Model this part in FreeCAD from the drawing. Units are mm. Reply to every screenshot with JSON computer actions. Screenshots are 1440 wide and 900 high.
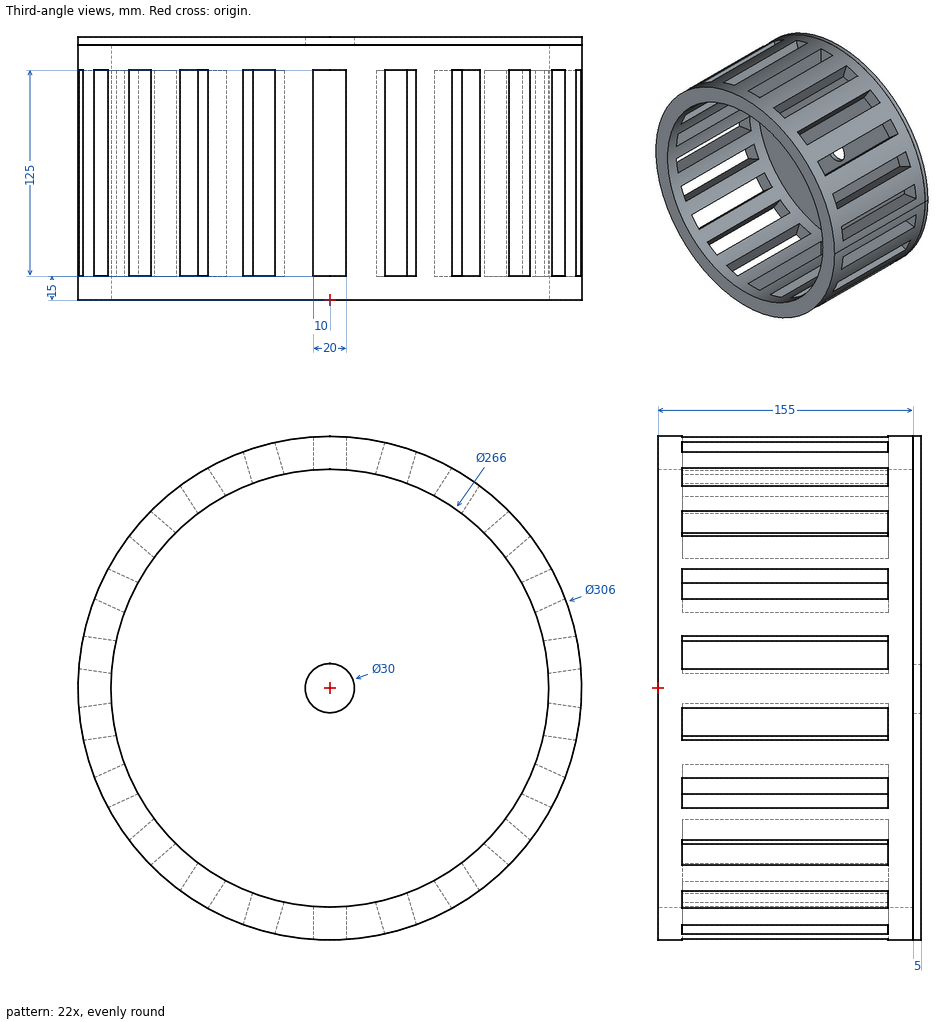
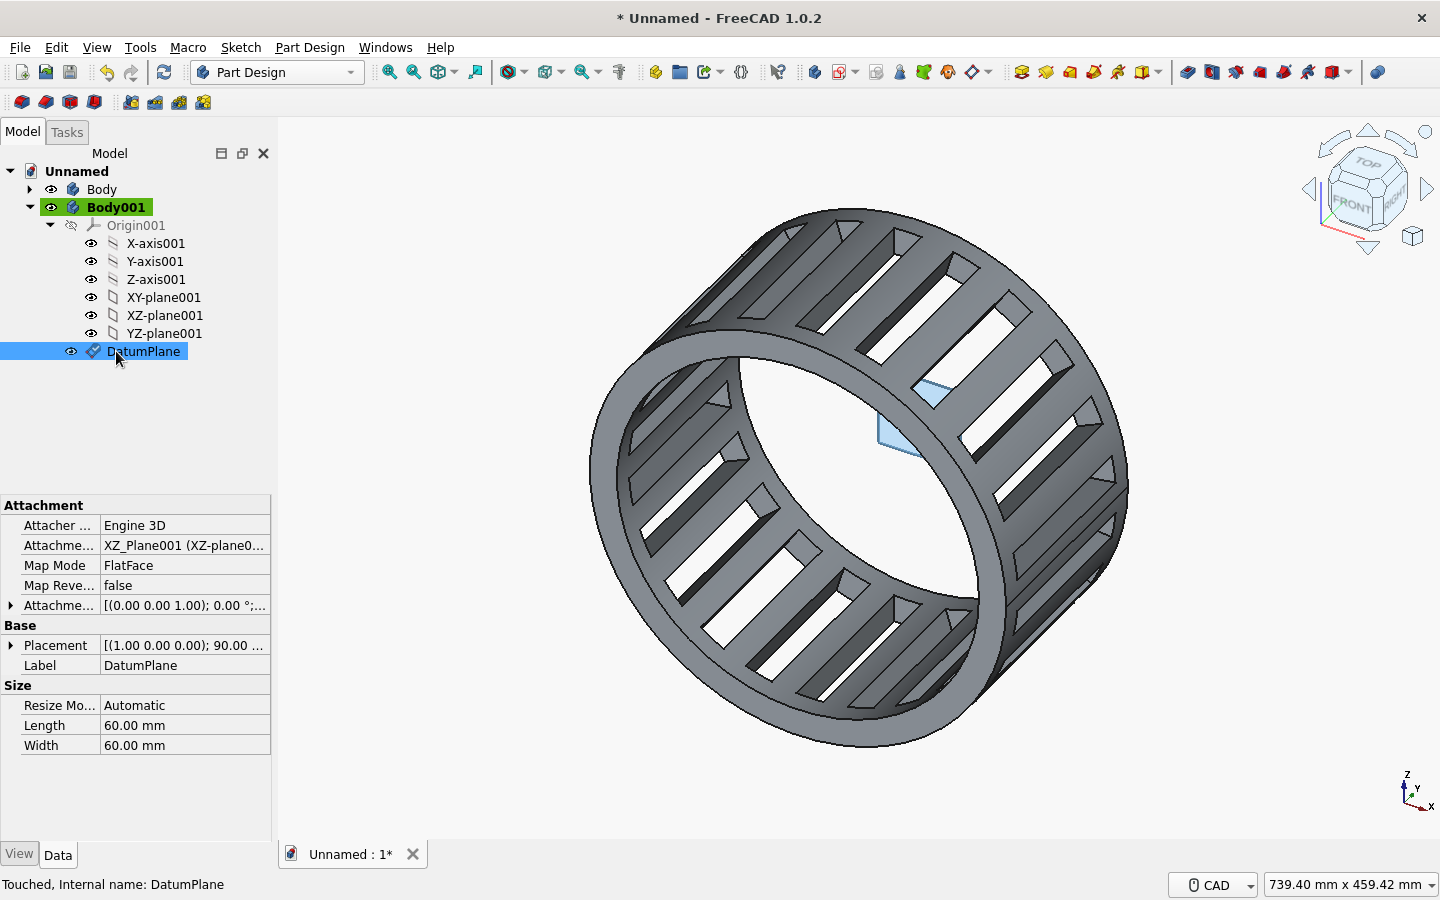
{"action": "left_click", "coordinate": [840, 72]}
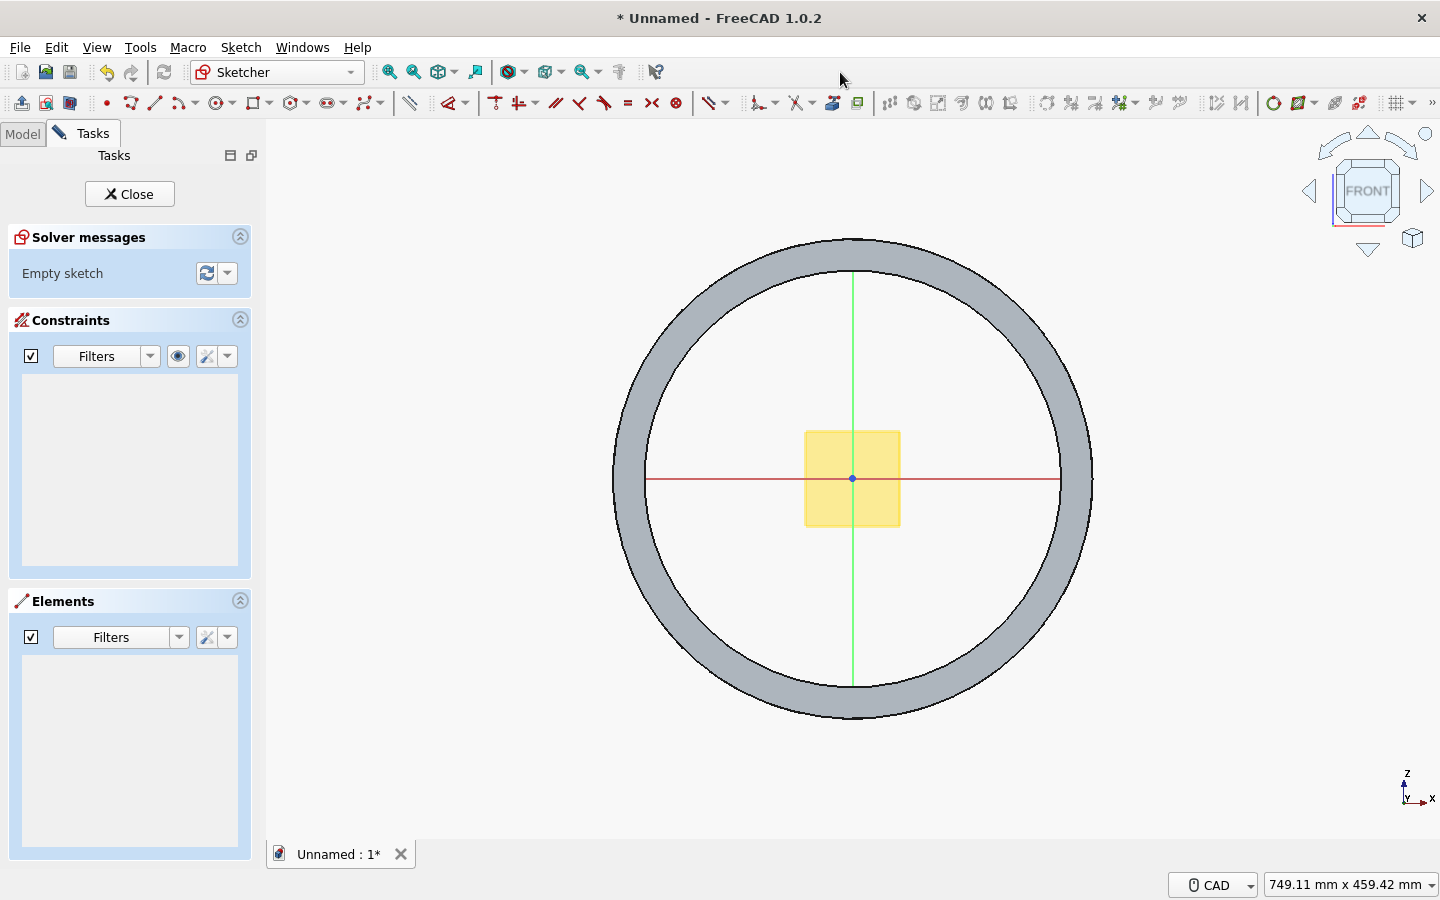
{"action": "left_click", "coordinate": [216, 104]}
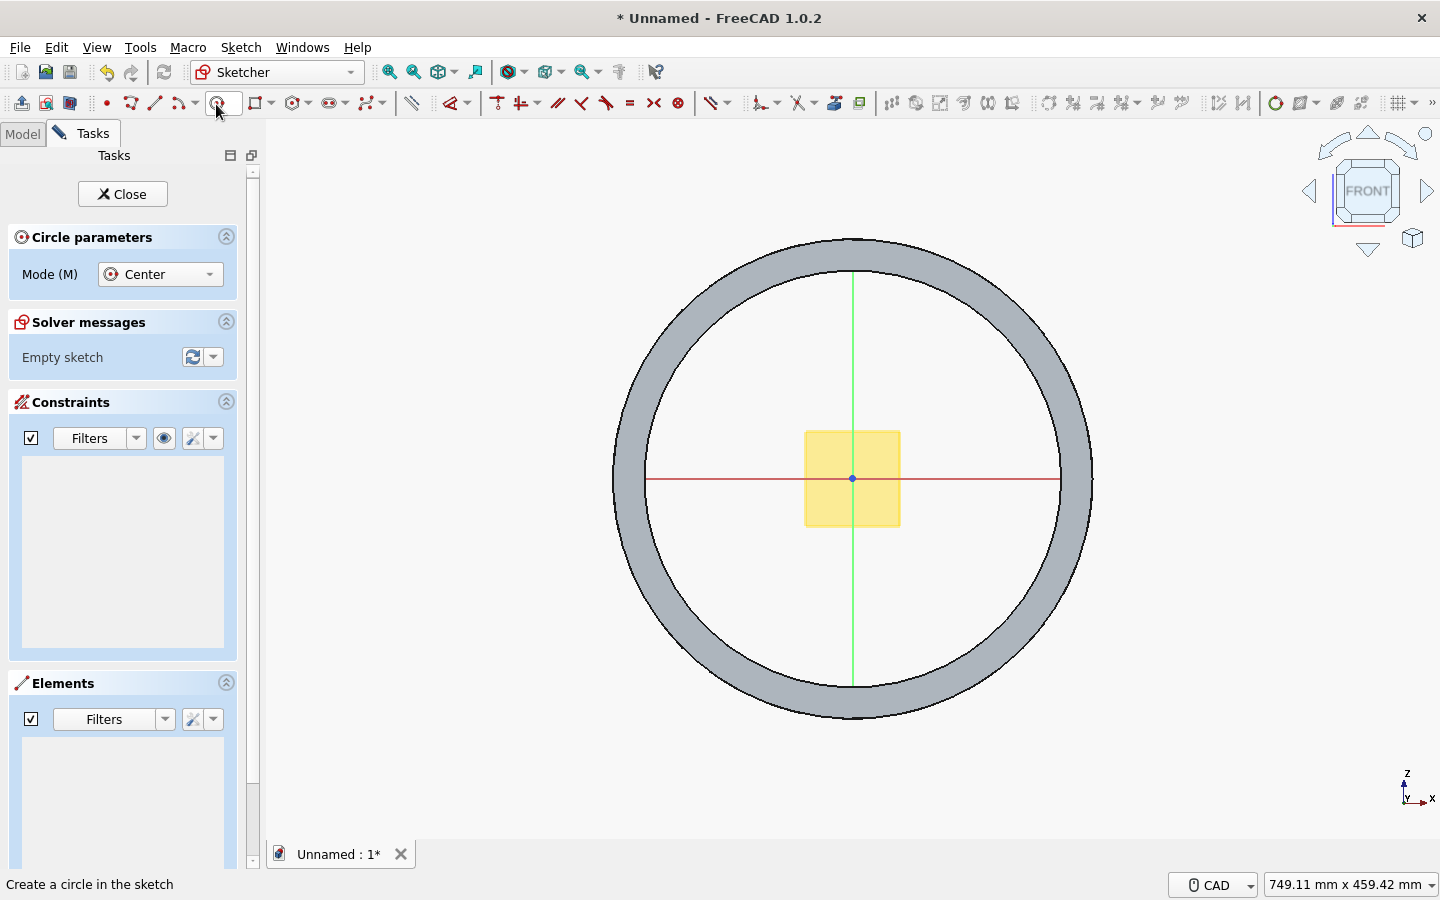
{"action": "left_click", "coordinate": [853, 479]}
{"action": "left_click", "coordinate": [1022, 309]}
{"action": "key", "text": "Escape"}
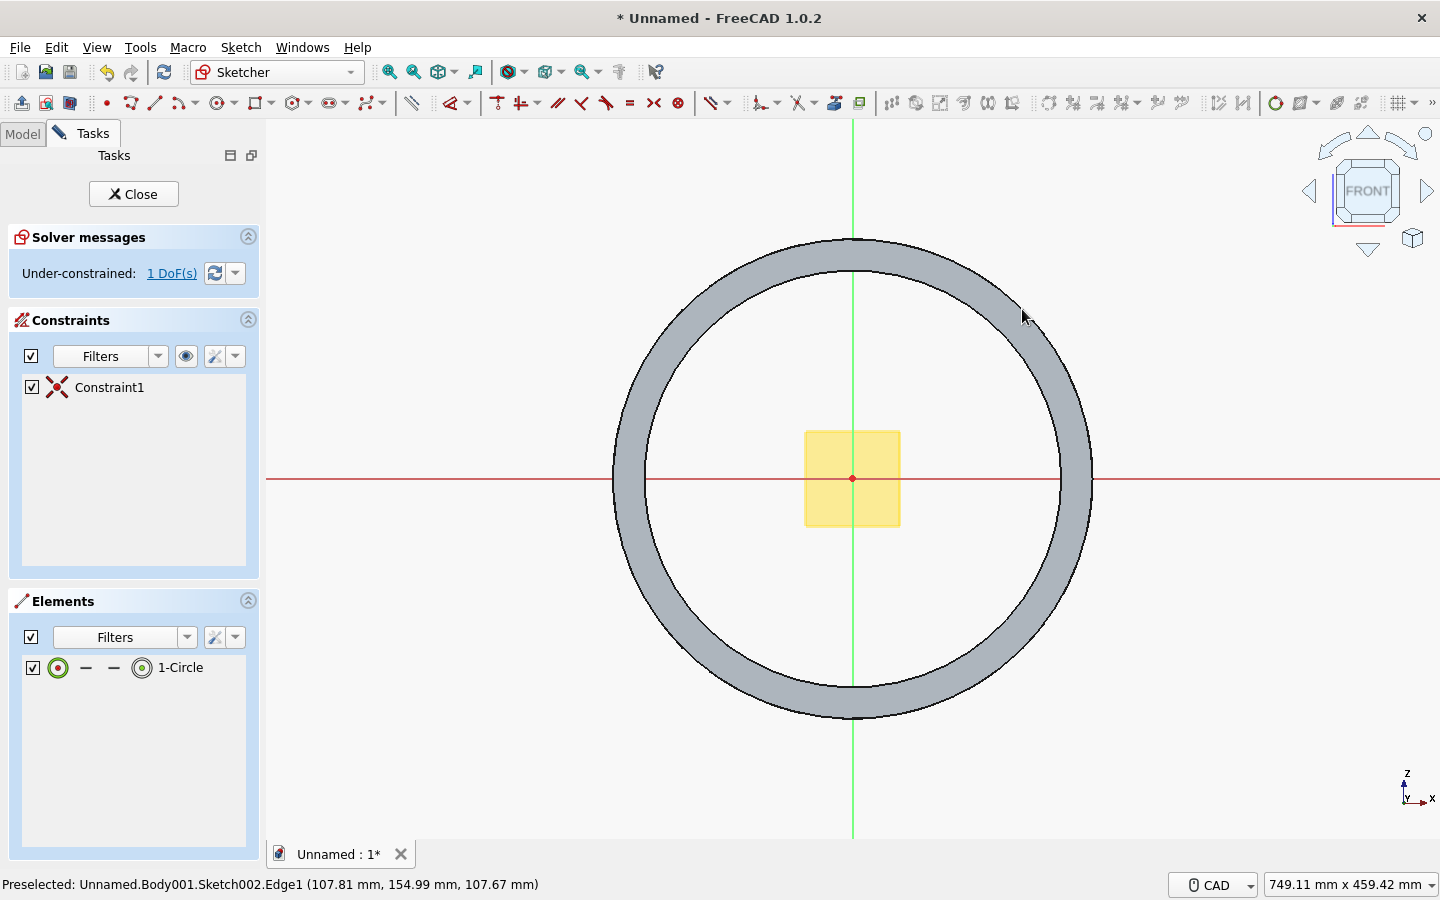
{"action": "left_click", "coordinate": [450, 104]}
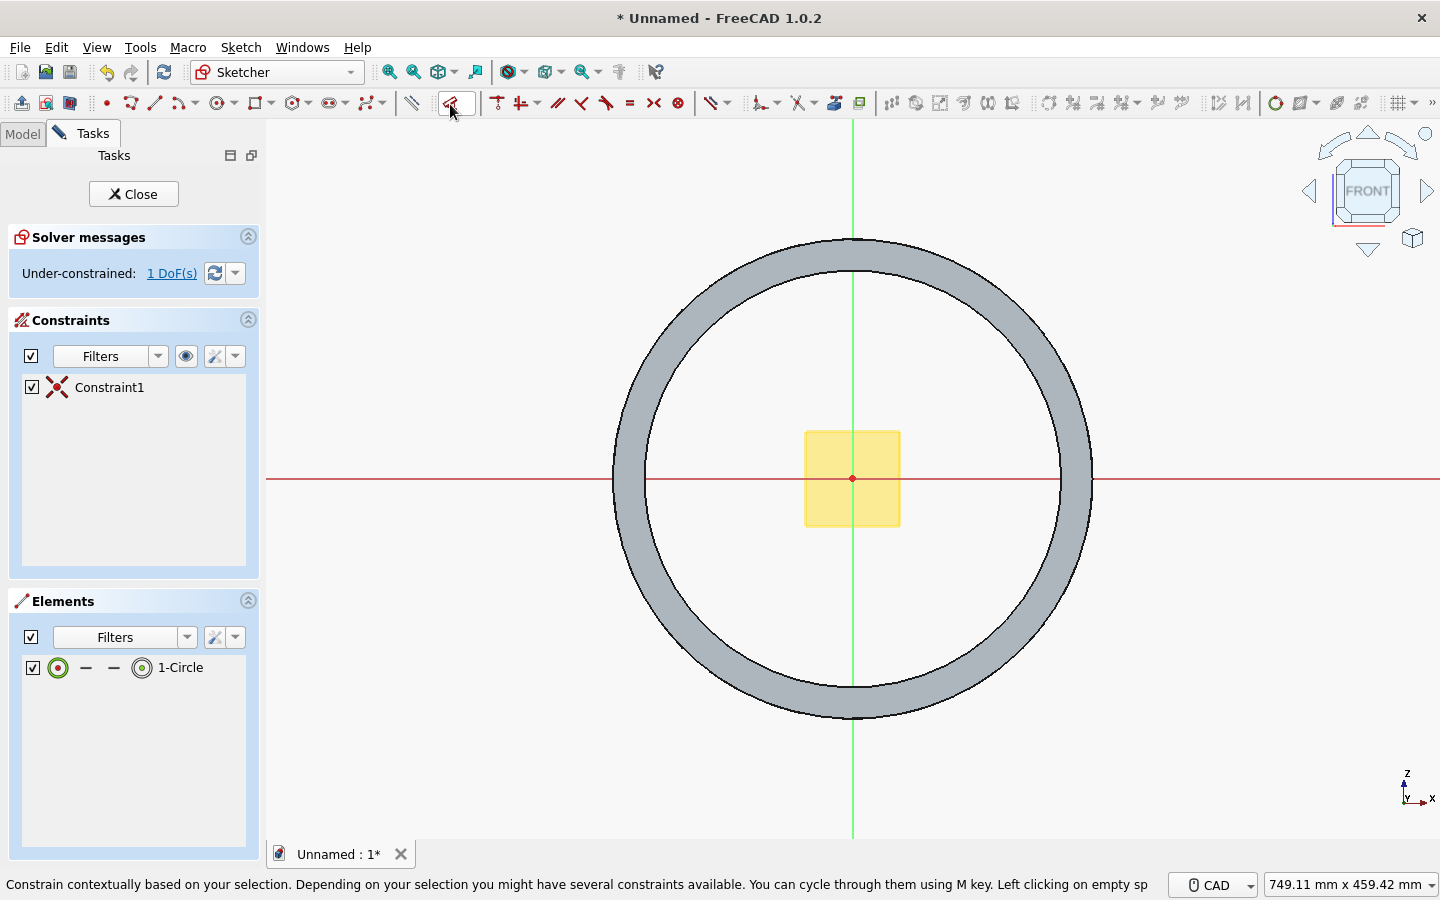
{"action": "left_click", "coordinate": [1021, 309]}
{"action": "left_click", "coordinate": [1044, 286]}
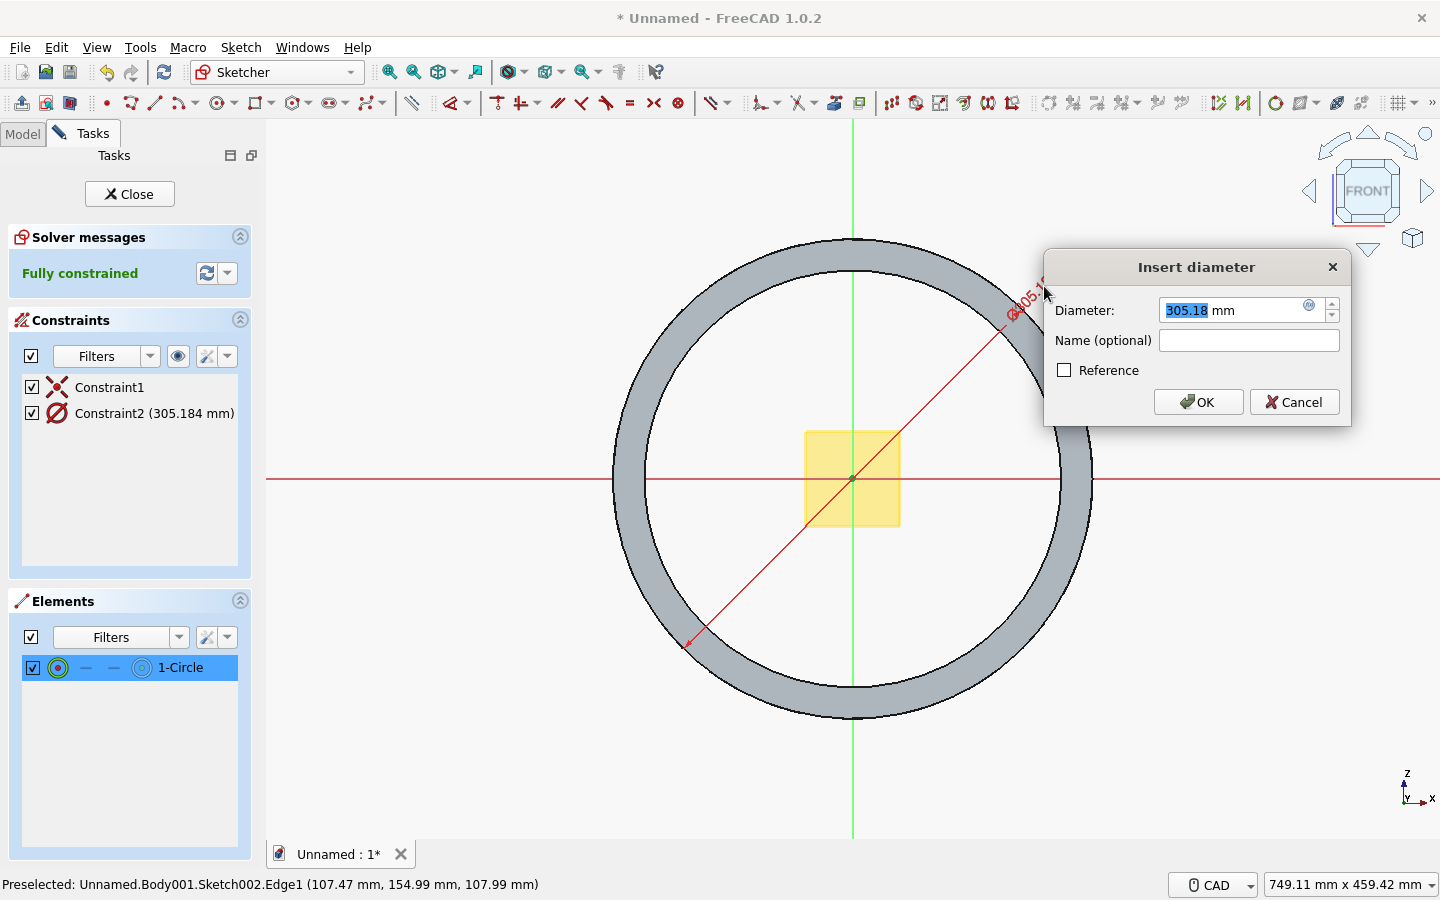
{"action": "type", "text": "306"}
{"action": "key", "text": "Return"}
{"action": "key", "text": "Escape"}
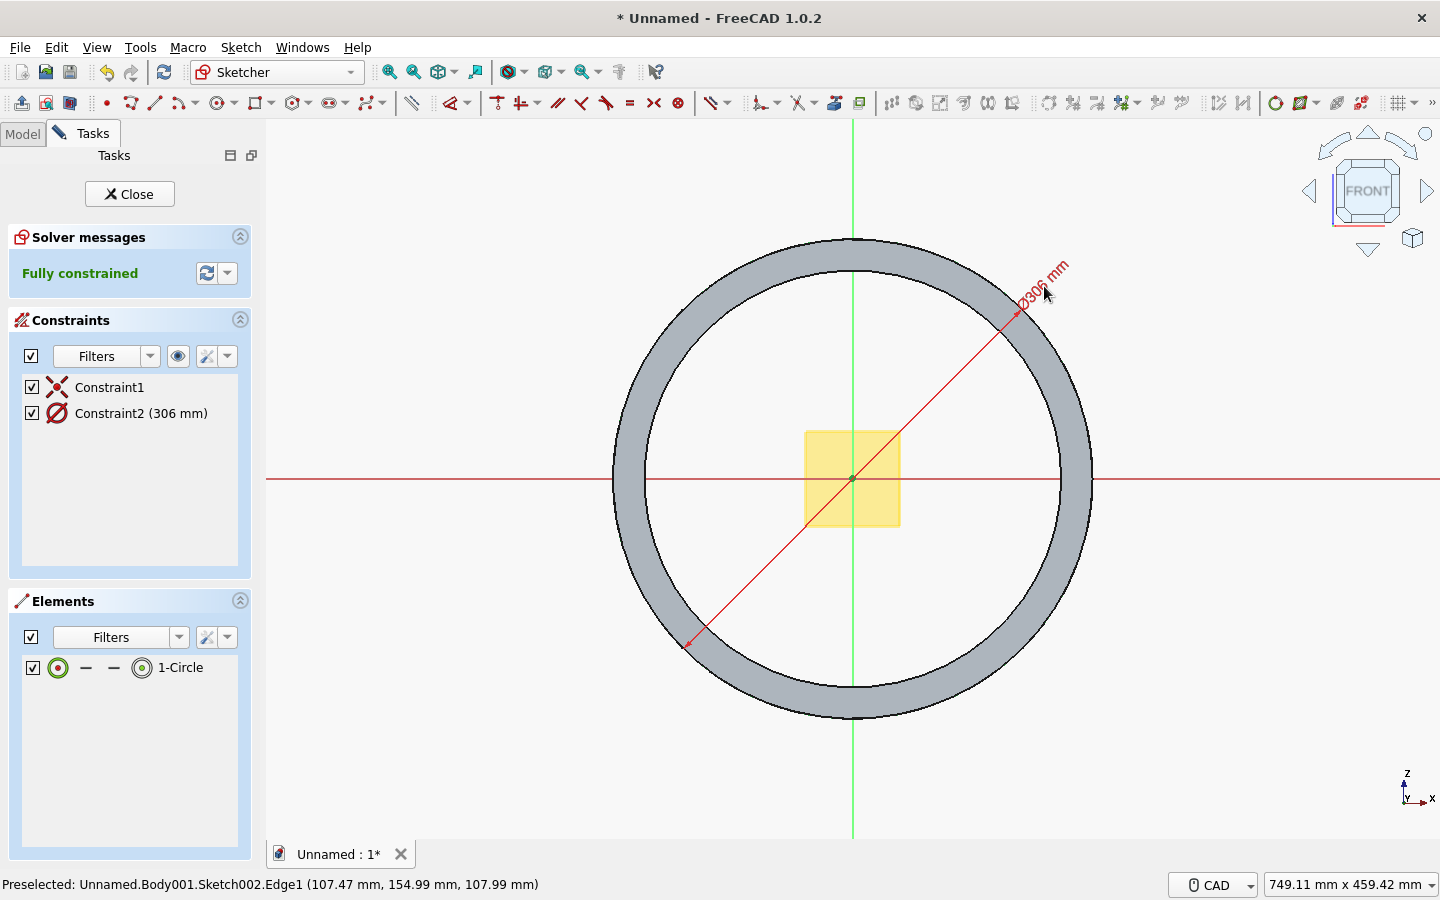
{"action": "left_click", "coordinate": [130, 194]}